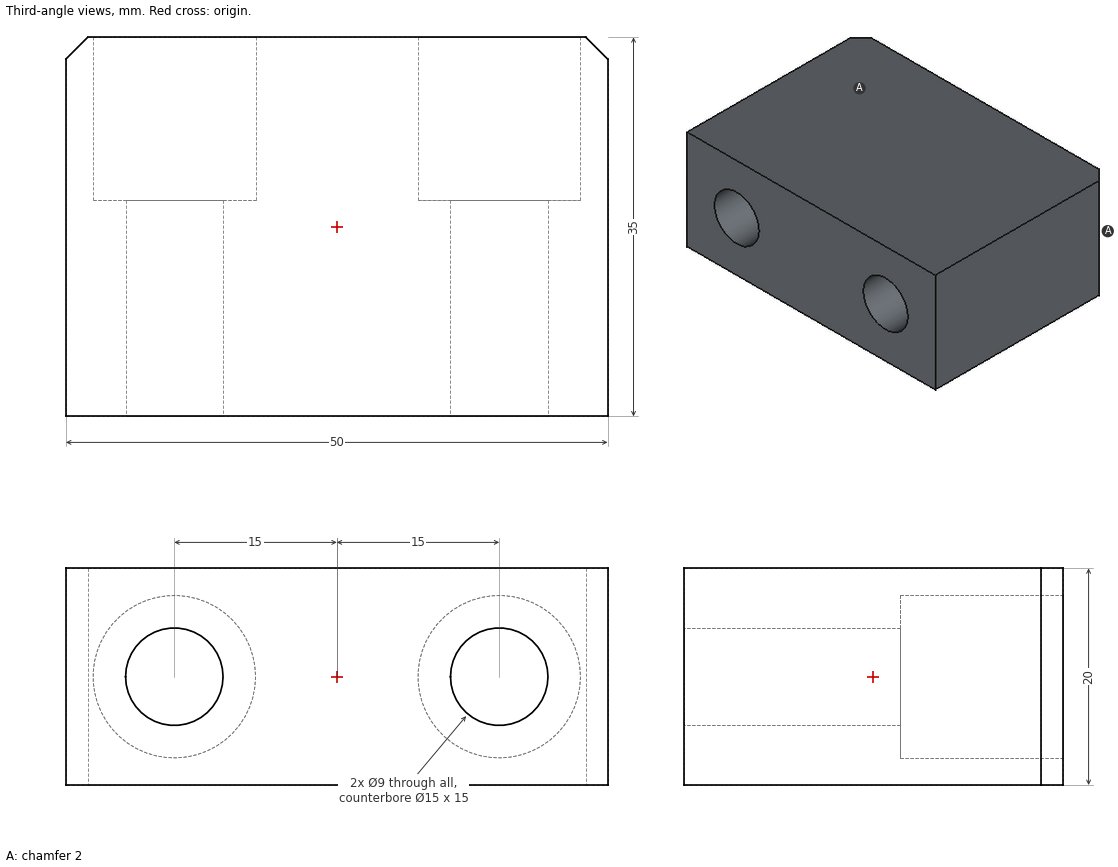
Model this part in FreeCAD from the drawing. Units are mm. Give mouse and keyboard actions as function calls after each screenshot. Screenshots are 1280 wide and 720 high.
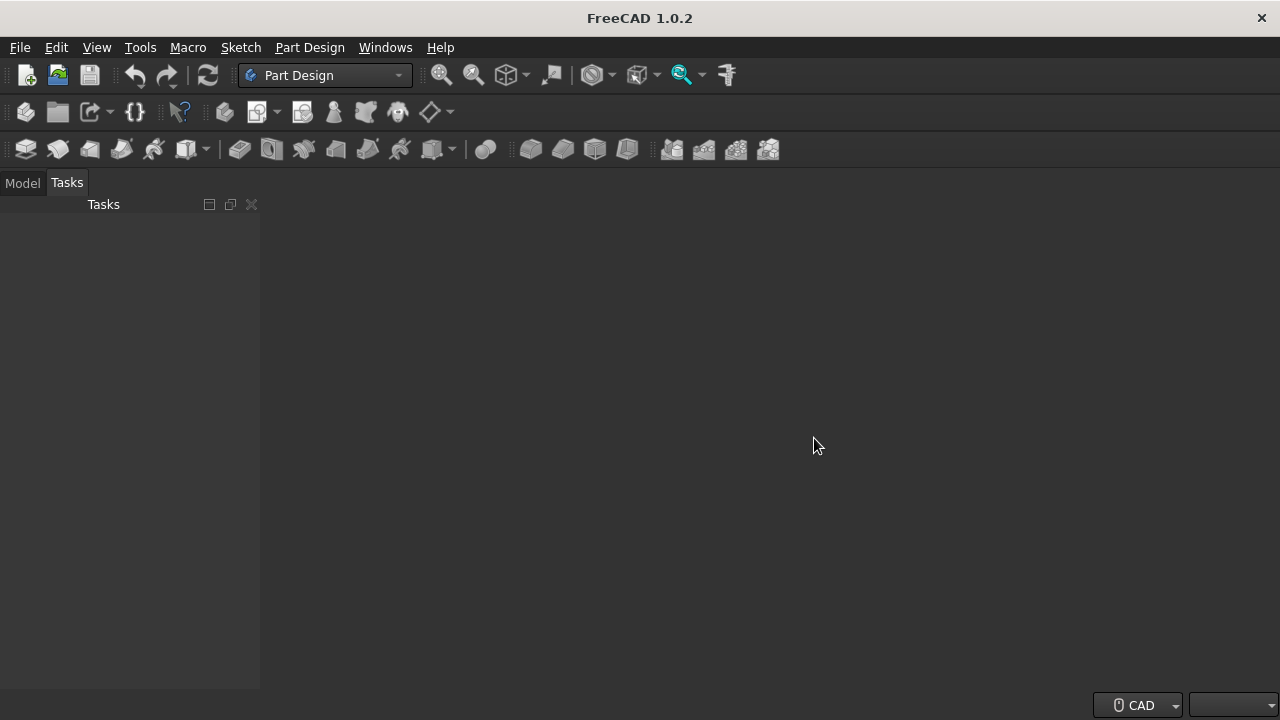
click(26, 76)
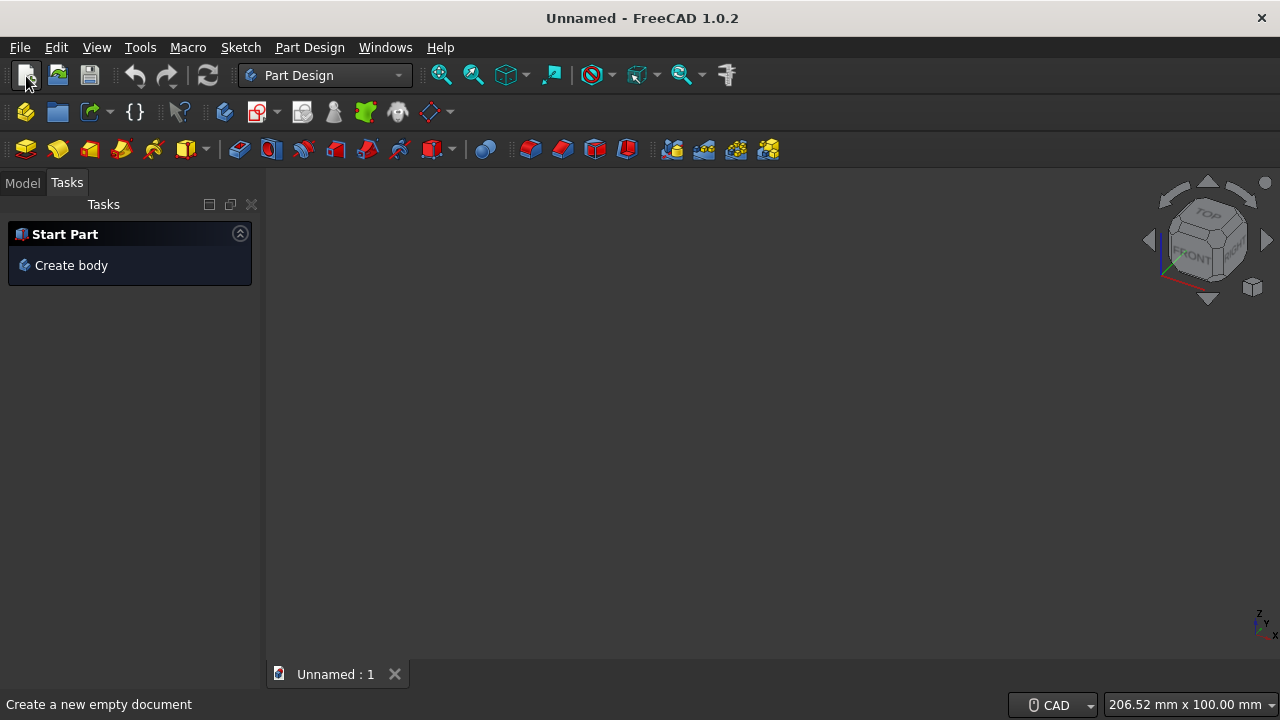
click(258, 112)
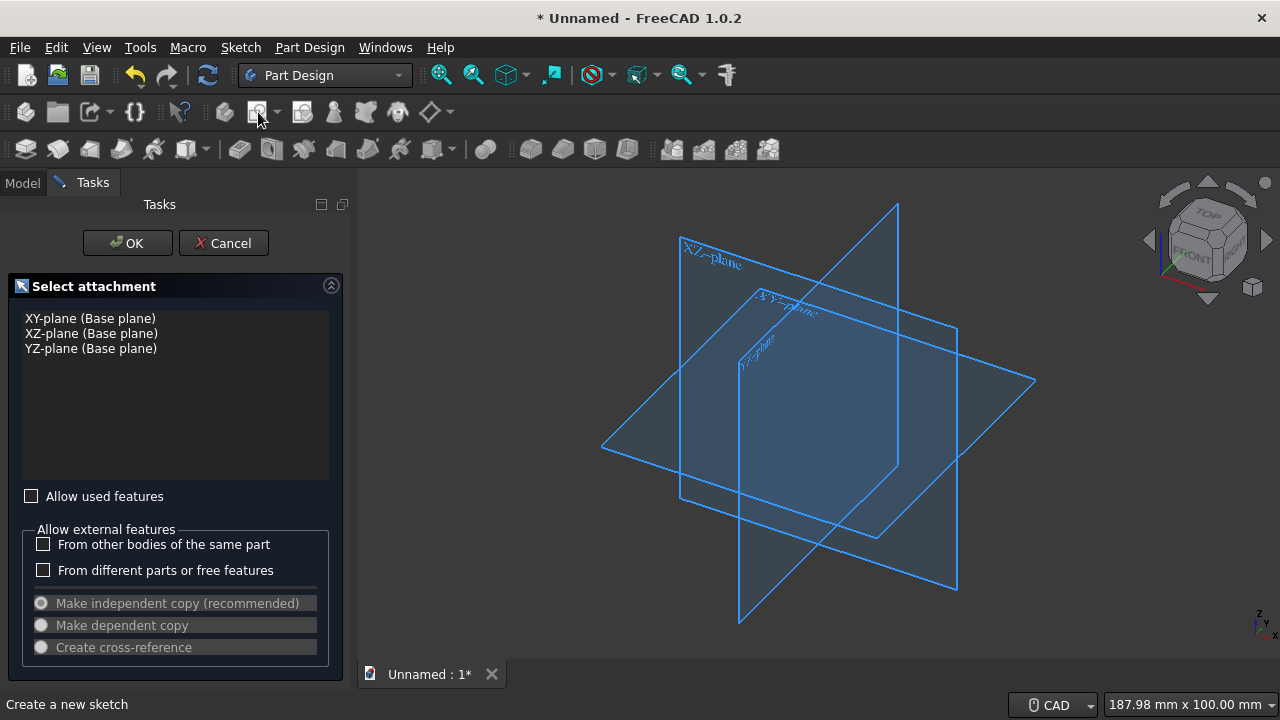
click(82, 318)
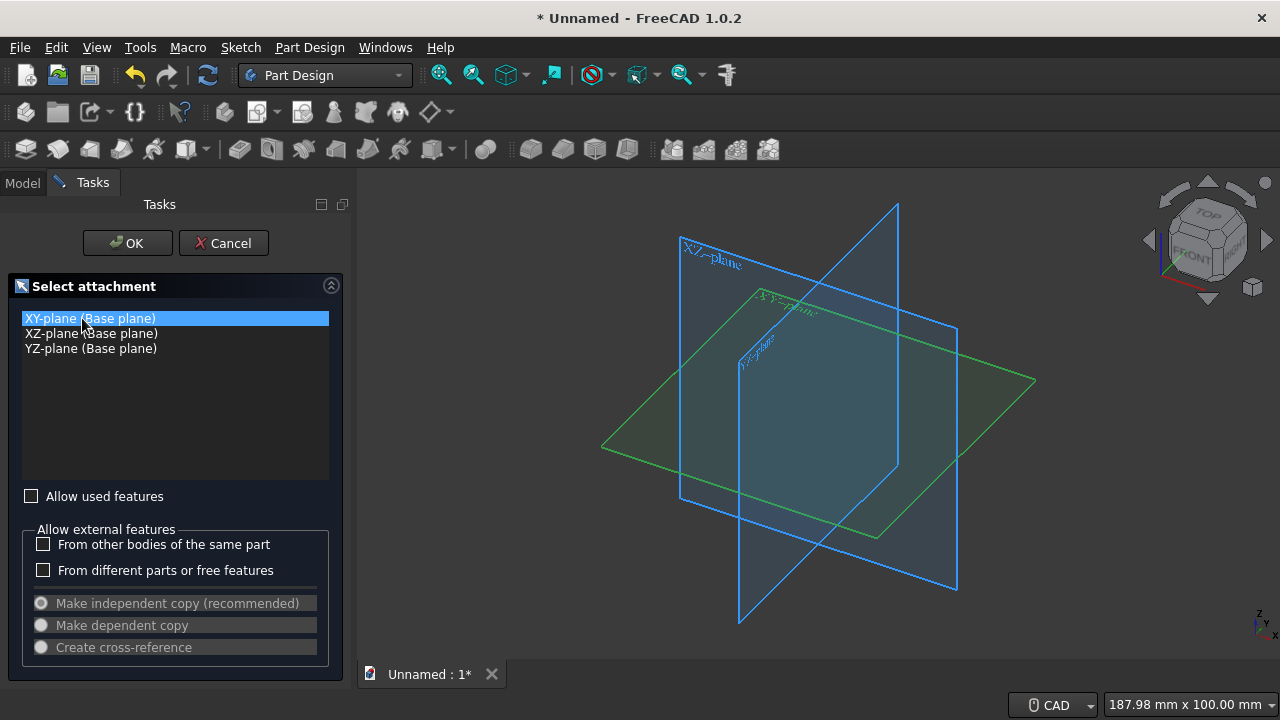
click(128, 243)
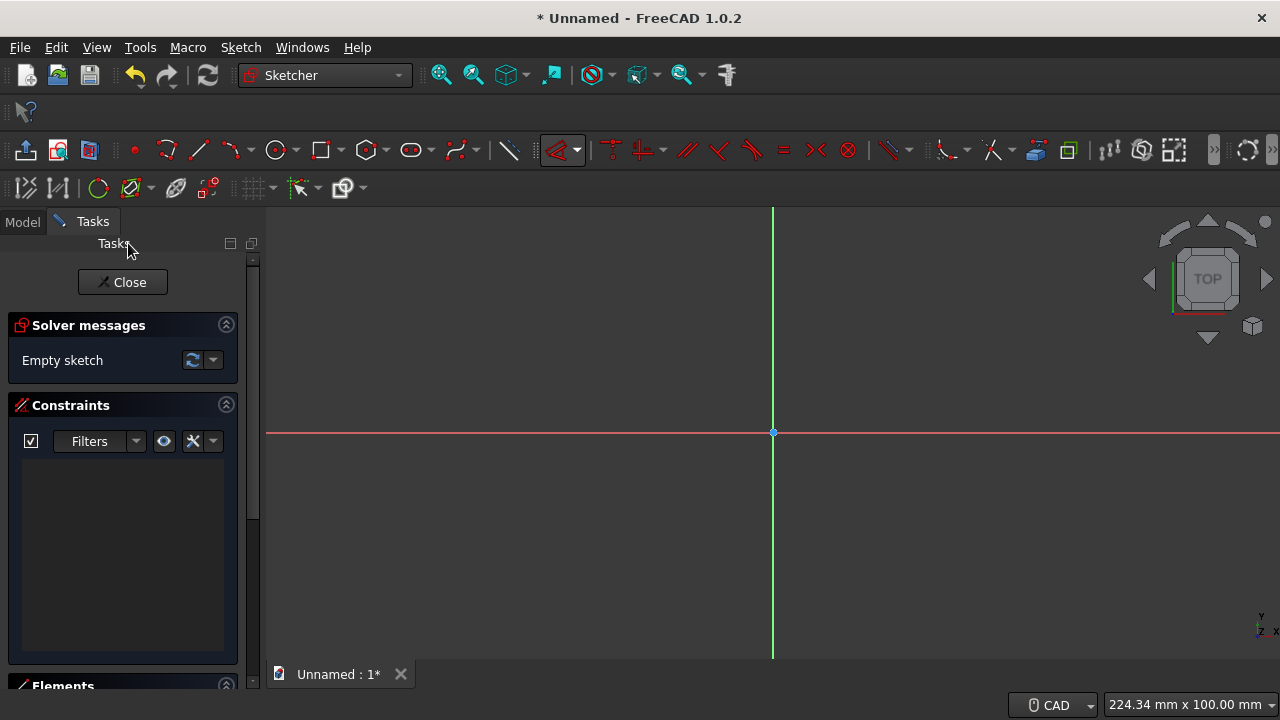
scroll(856, 433, up, 3)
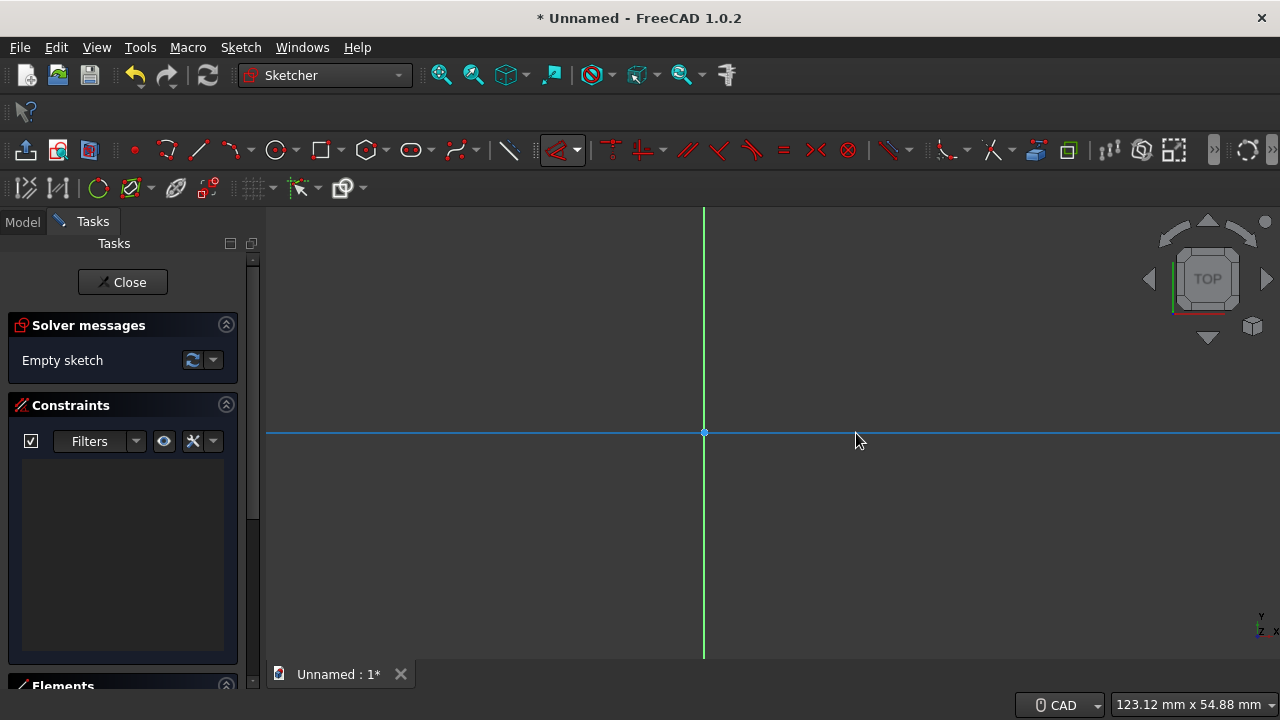
click(344, 150)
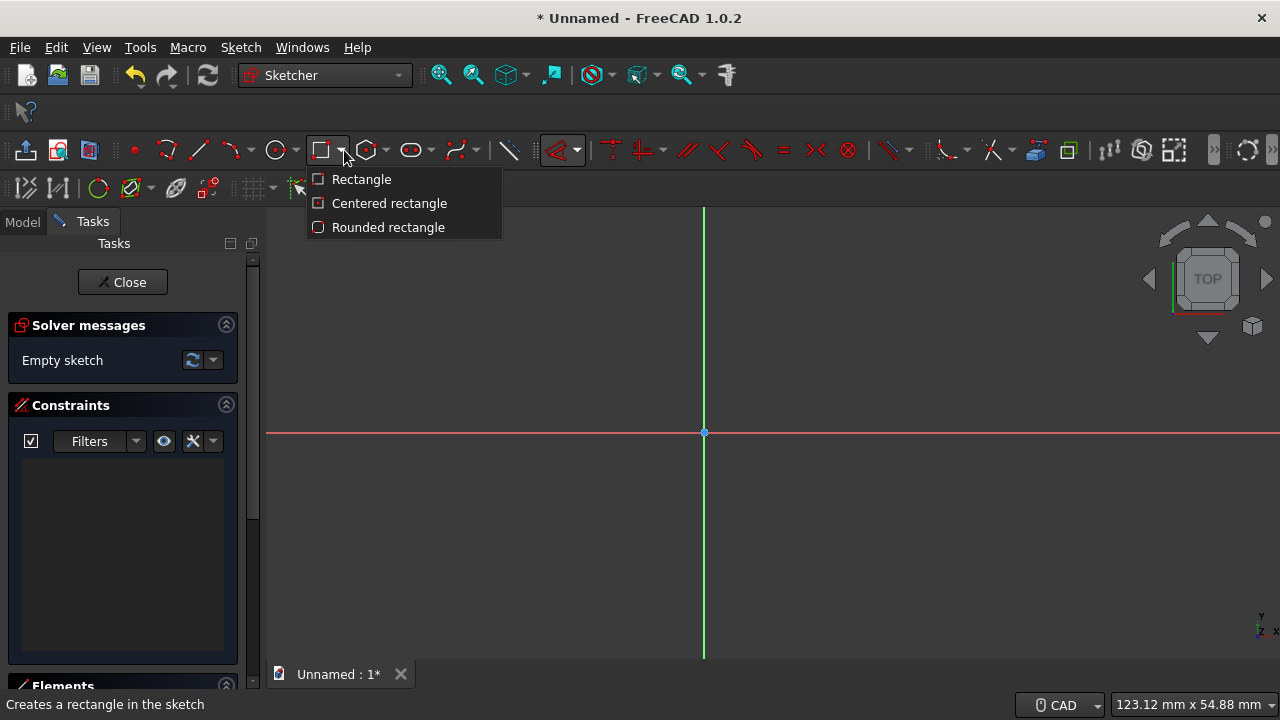
click(404, 203)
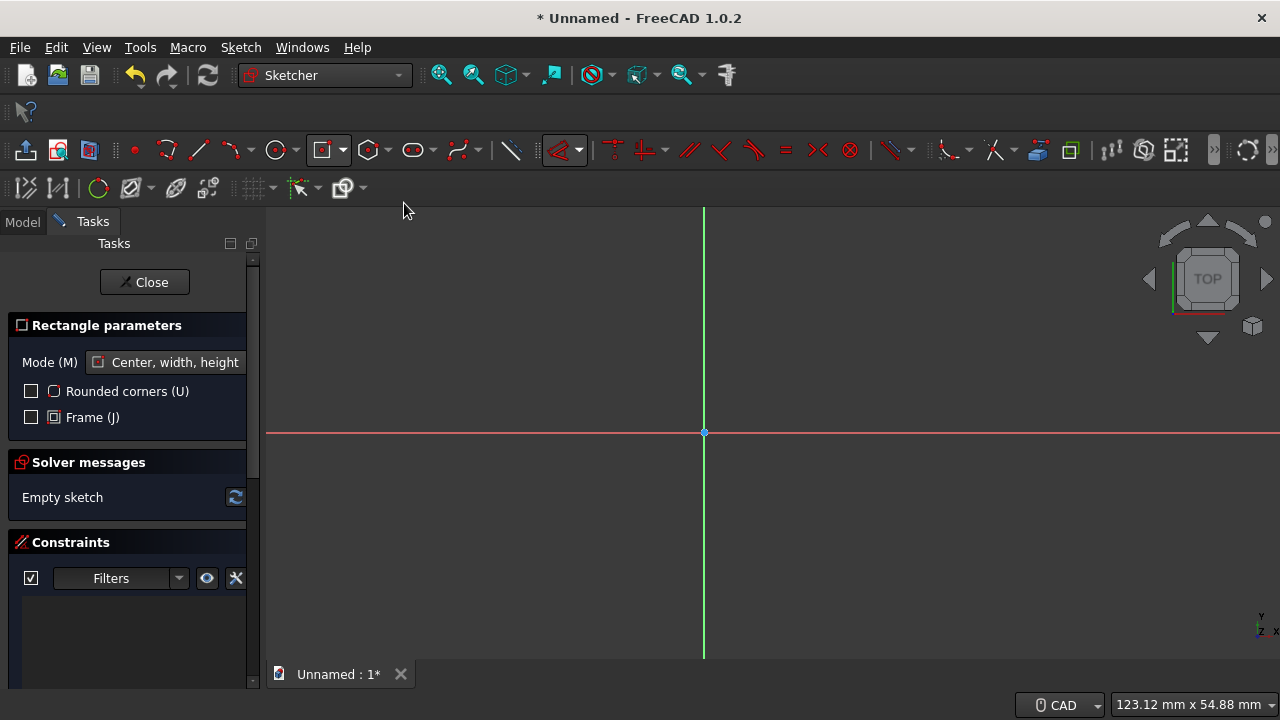
click(704, 433)
click(910, 288)
key(Escape)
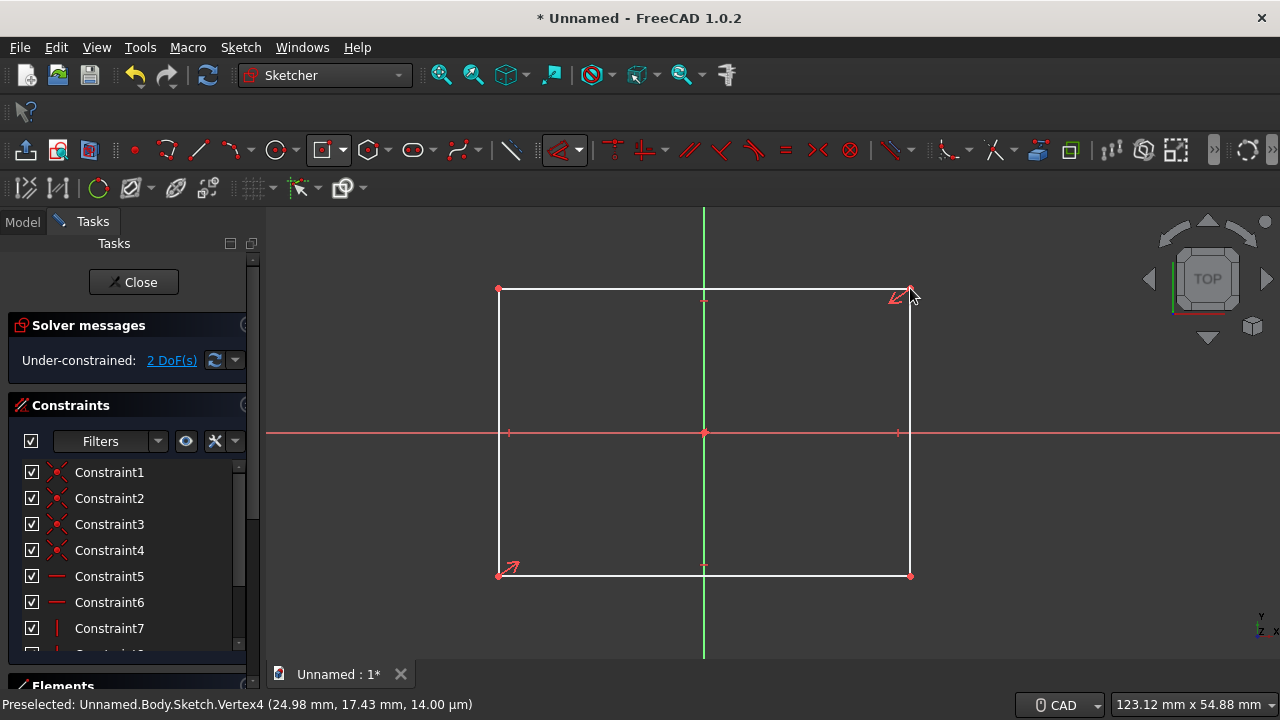
click(558, 150)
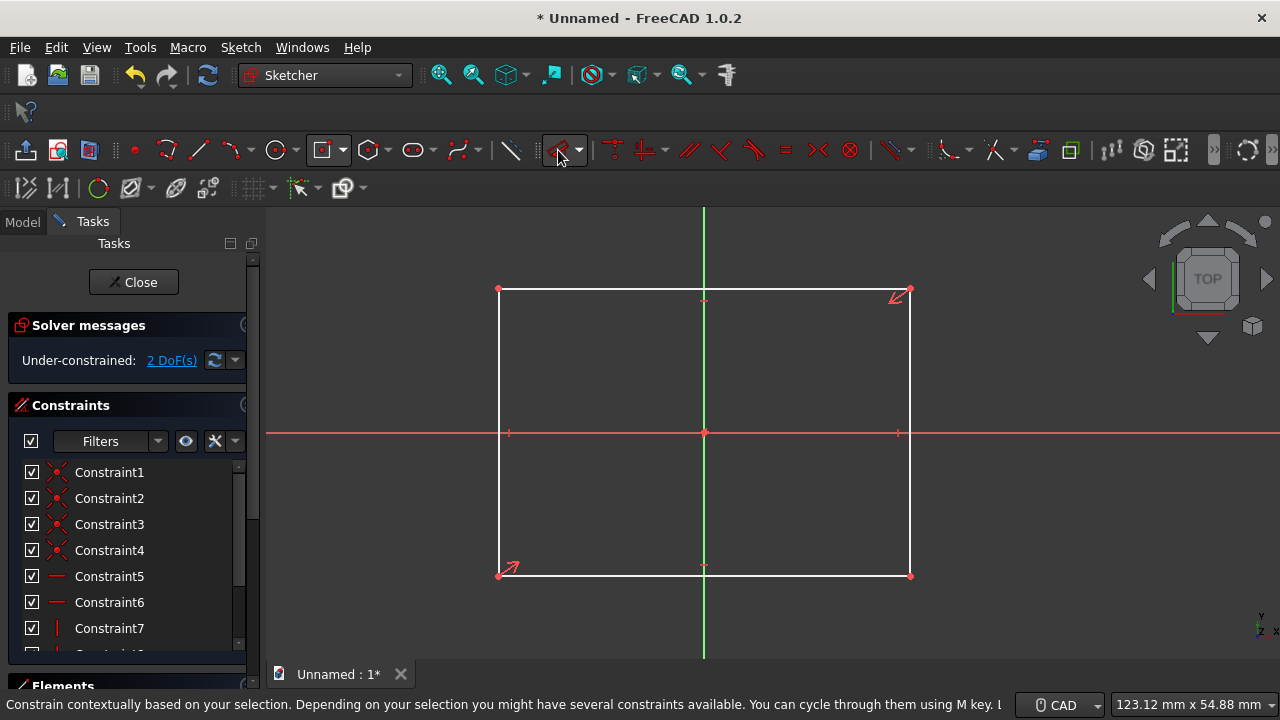
click(622, 576)
click(610, 610)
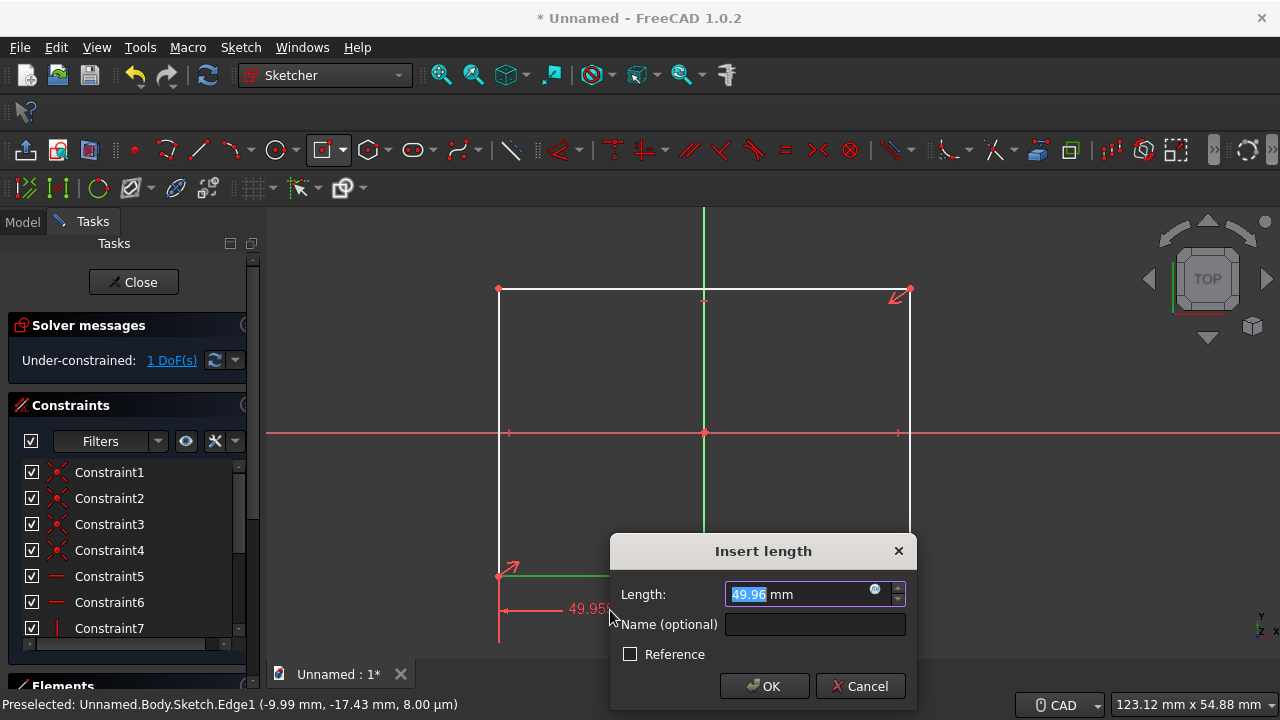
text(50)
key(Return)